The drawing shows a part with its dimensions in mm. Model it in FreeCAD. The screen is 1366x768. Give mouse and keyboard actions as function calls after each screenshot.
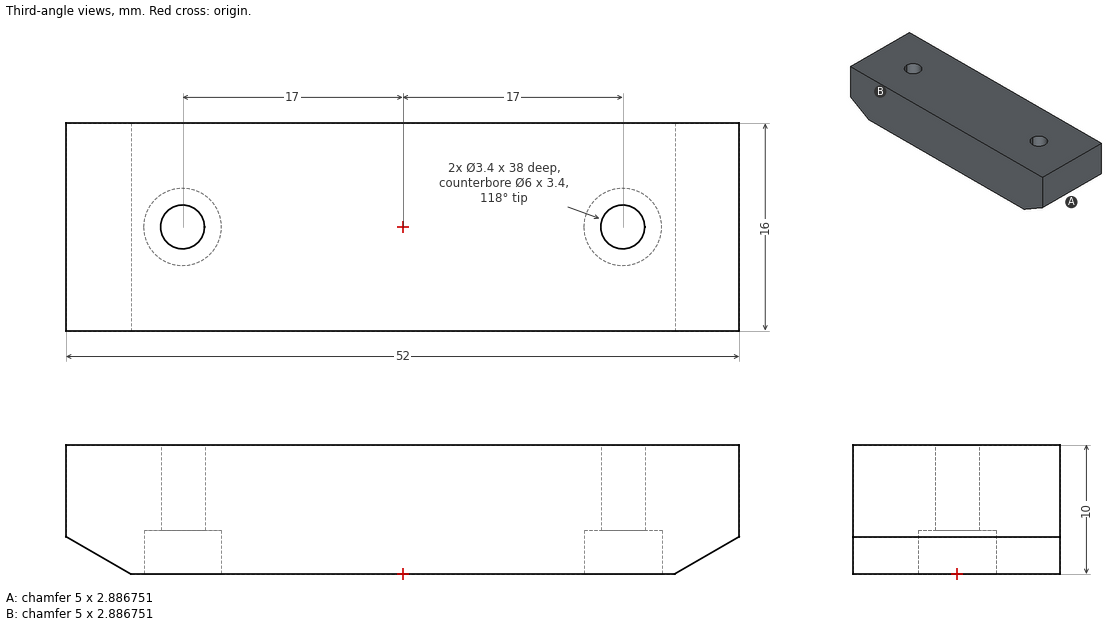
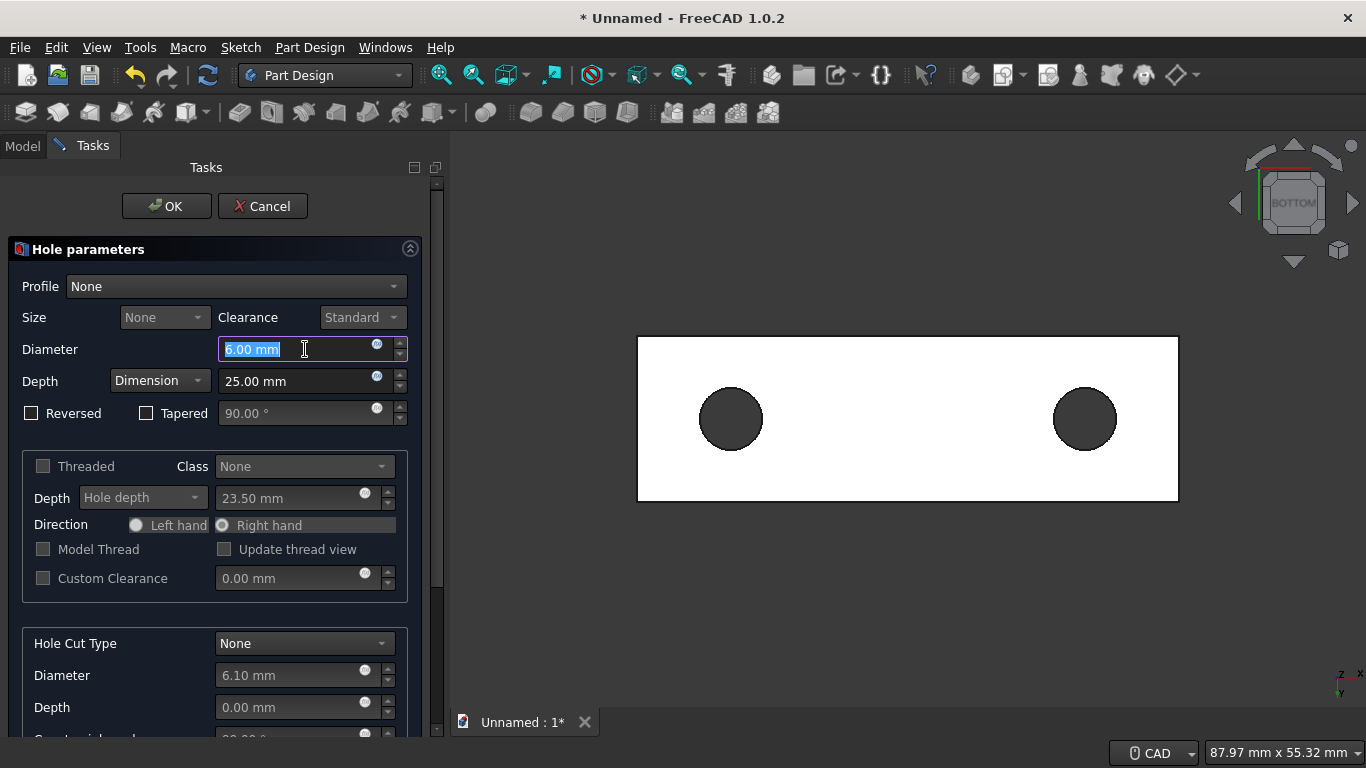
text(3.4)
key(Tab)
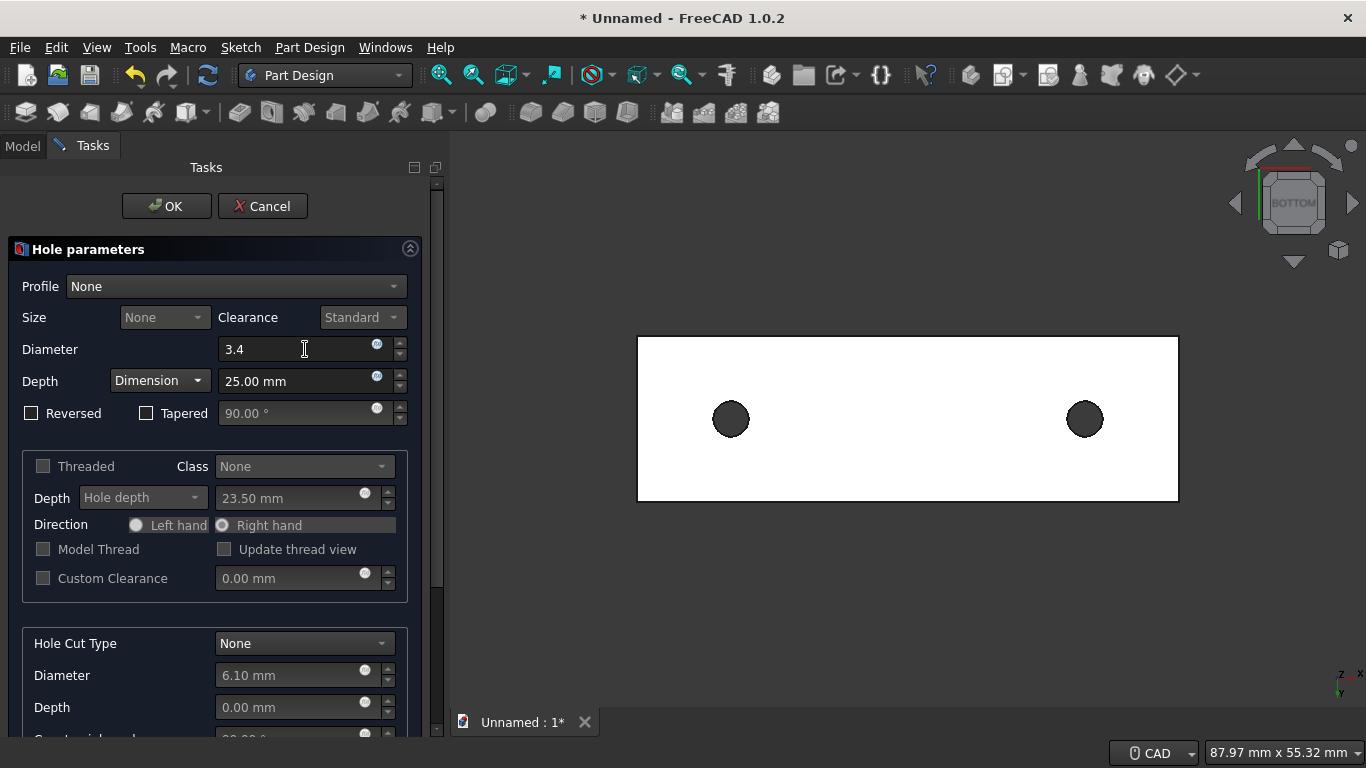
triple_click(305, 381)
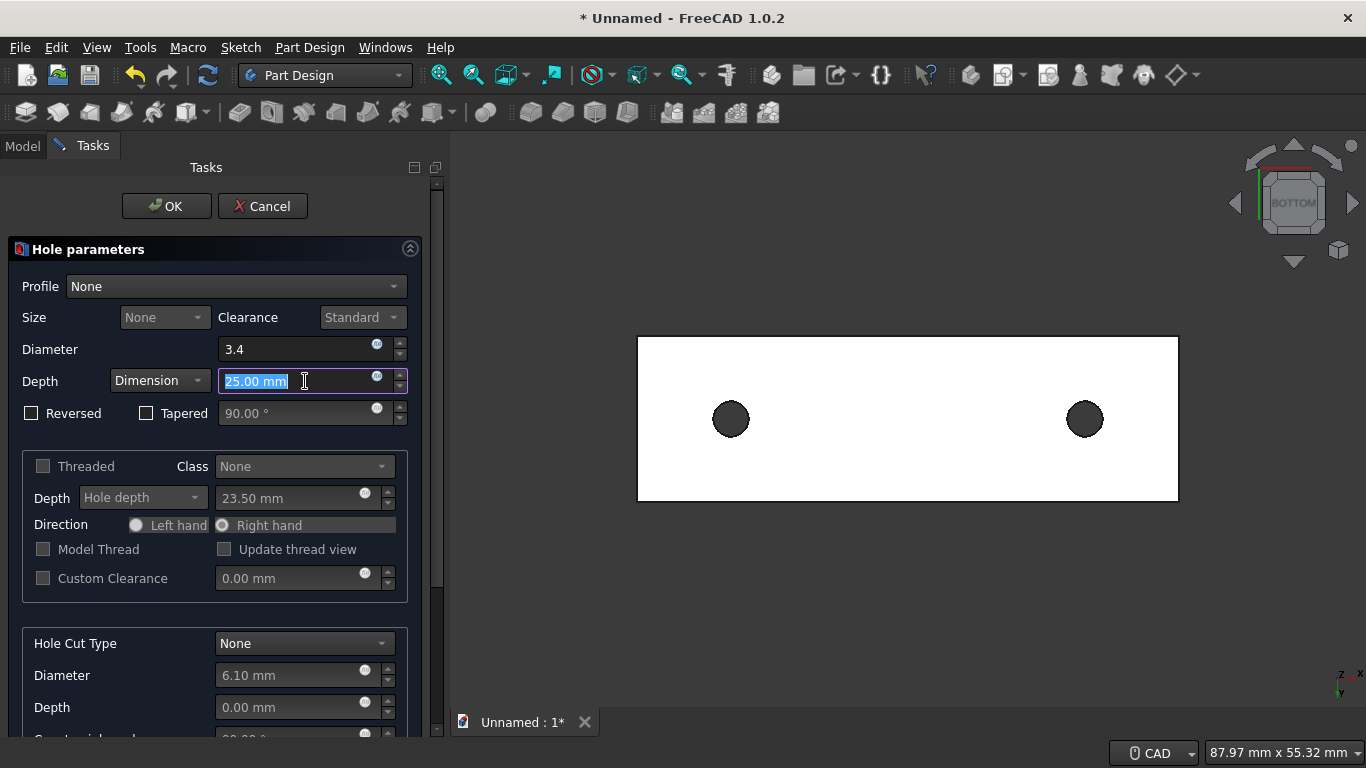
text(38)
key(Tab)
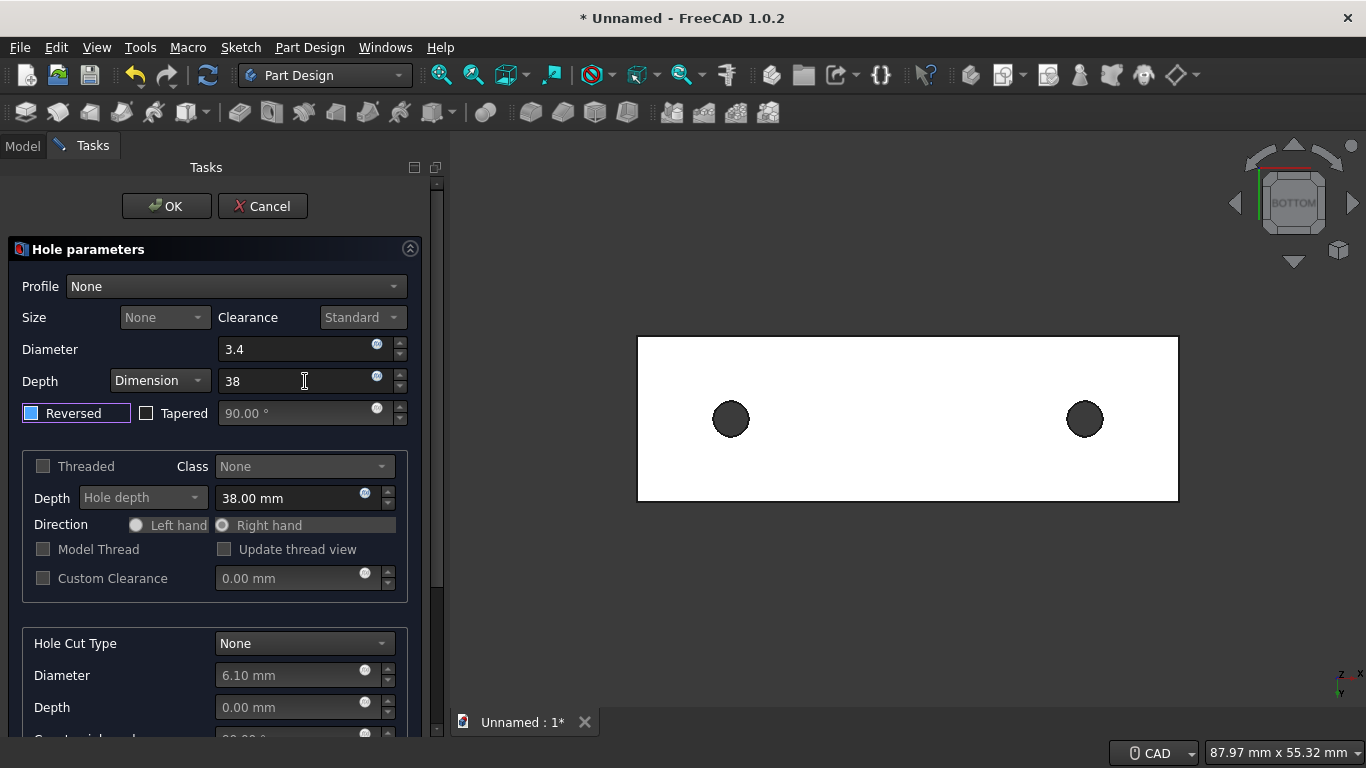
click(306, 644)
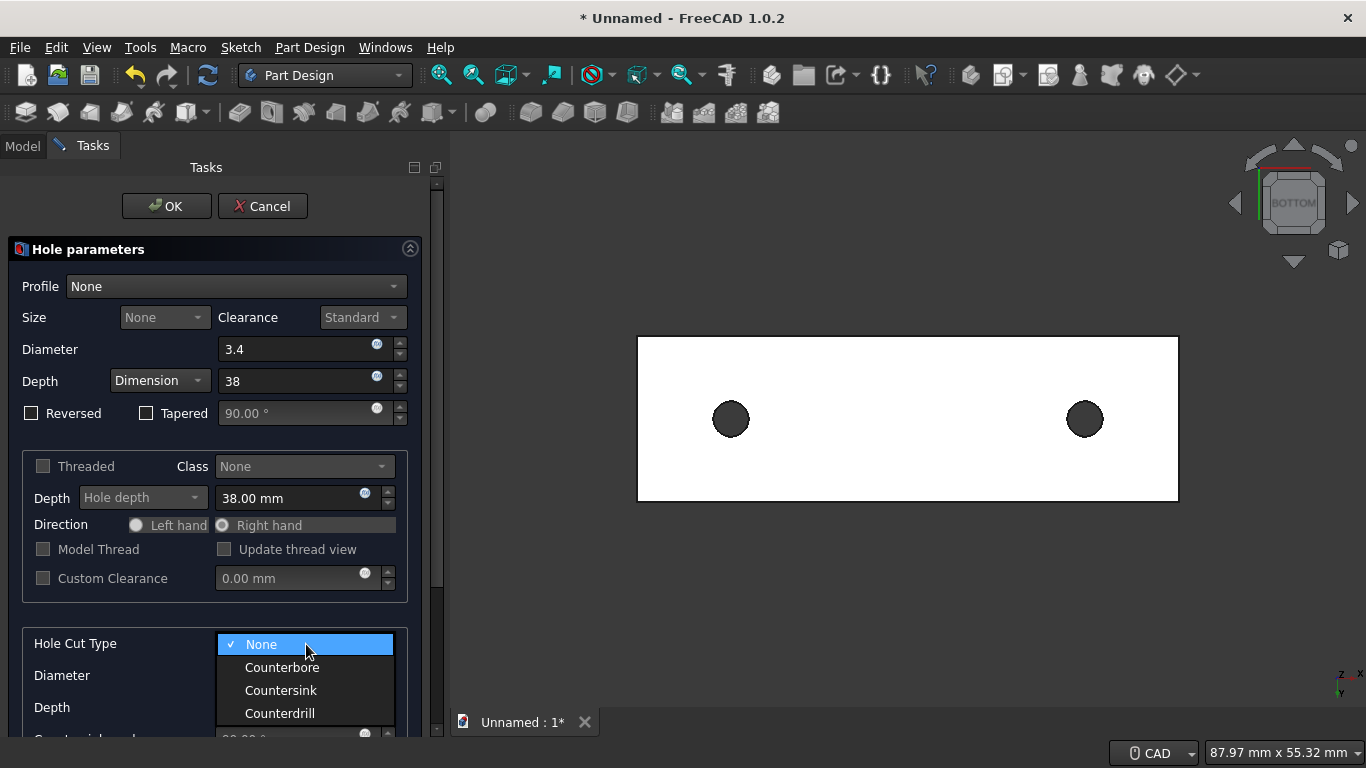
click(304, 668)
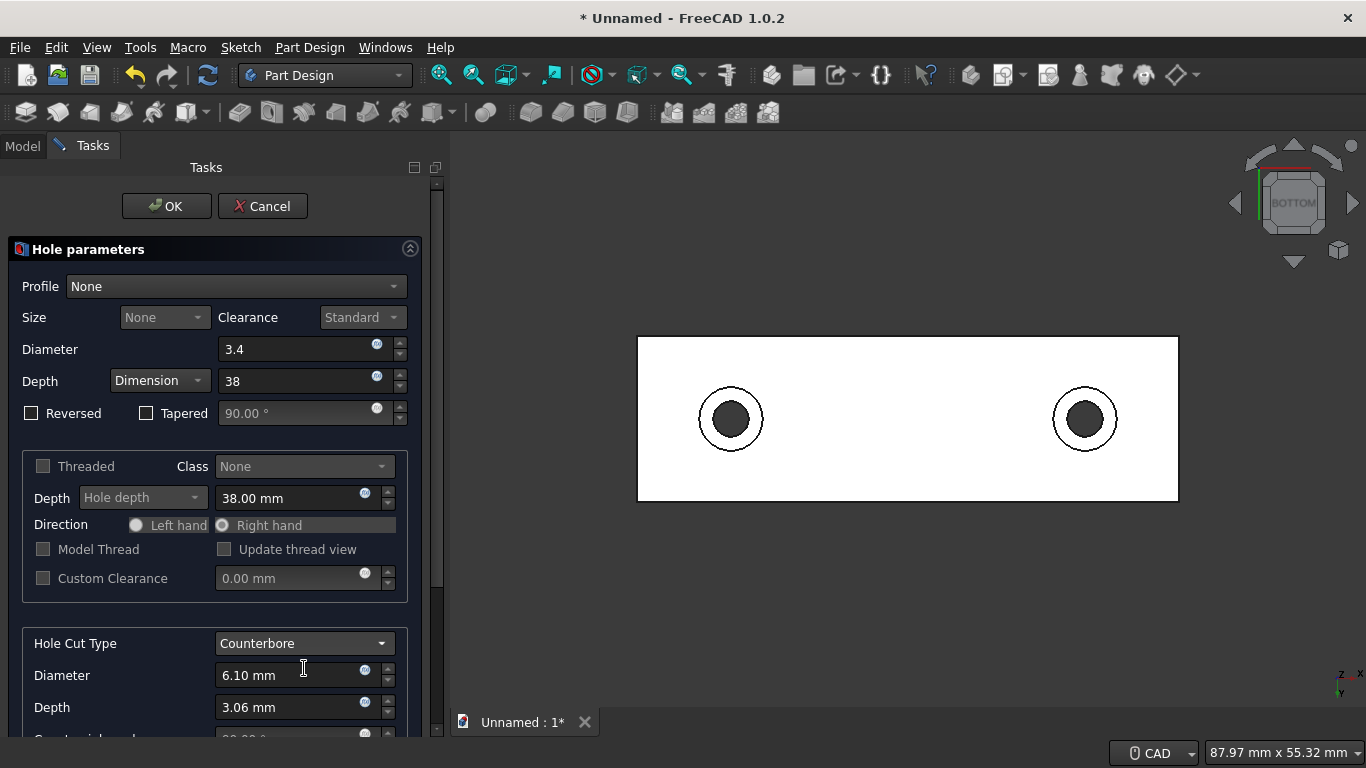
triple_click(298, 675)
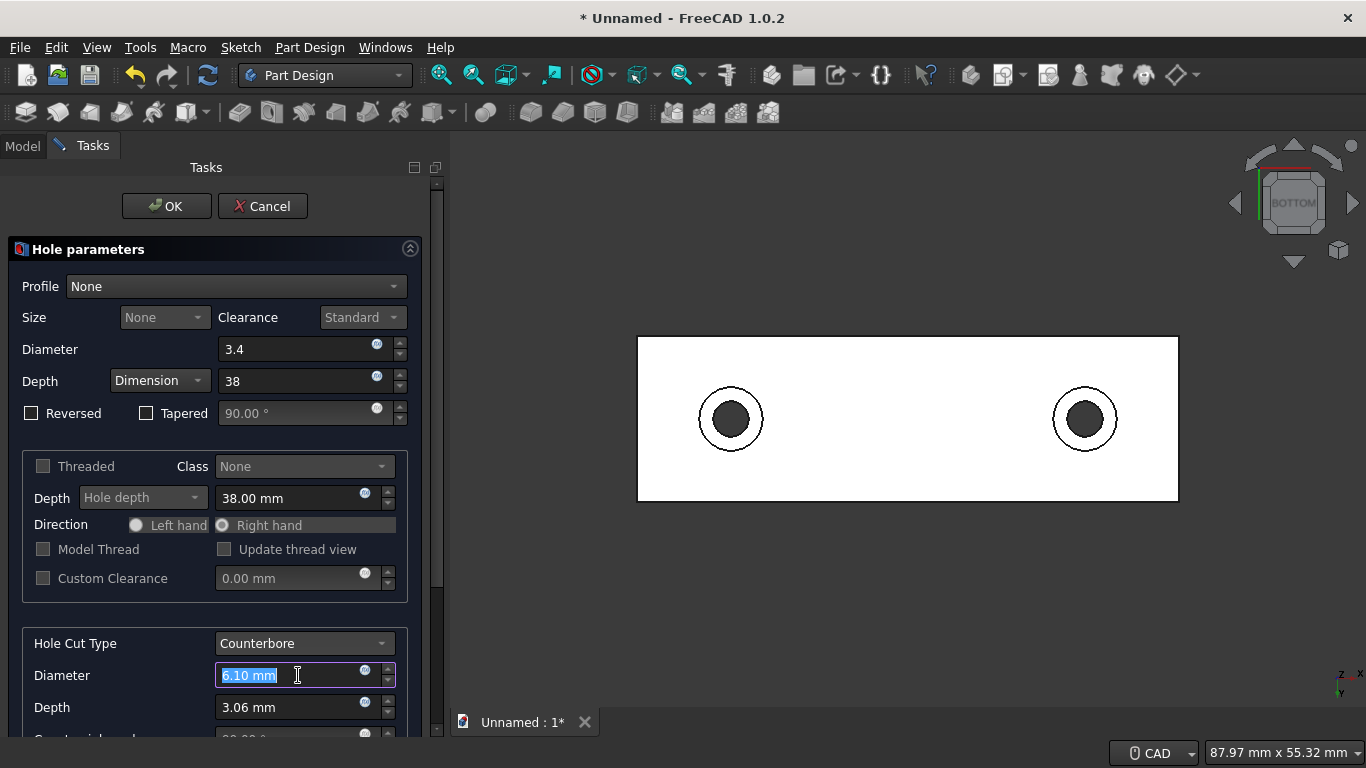
text(6)
key(Tab)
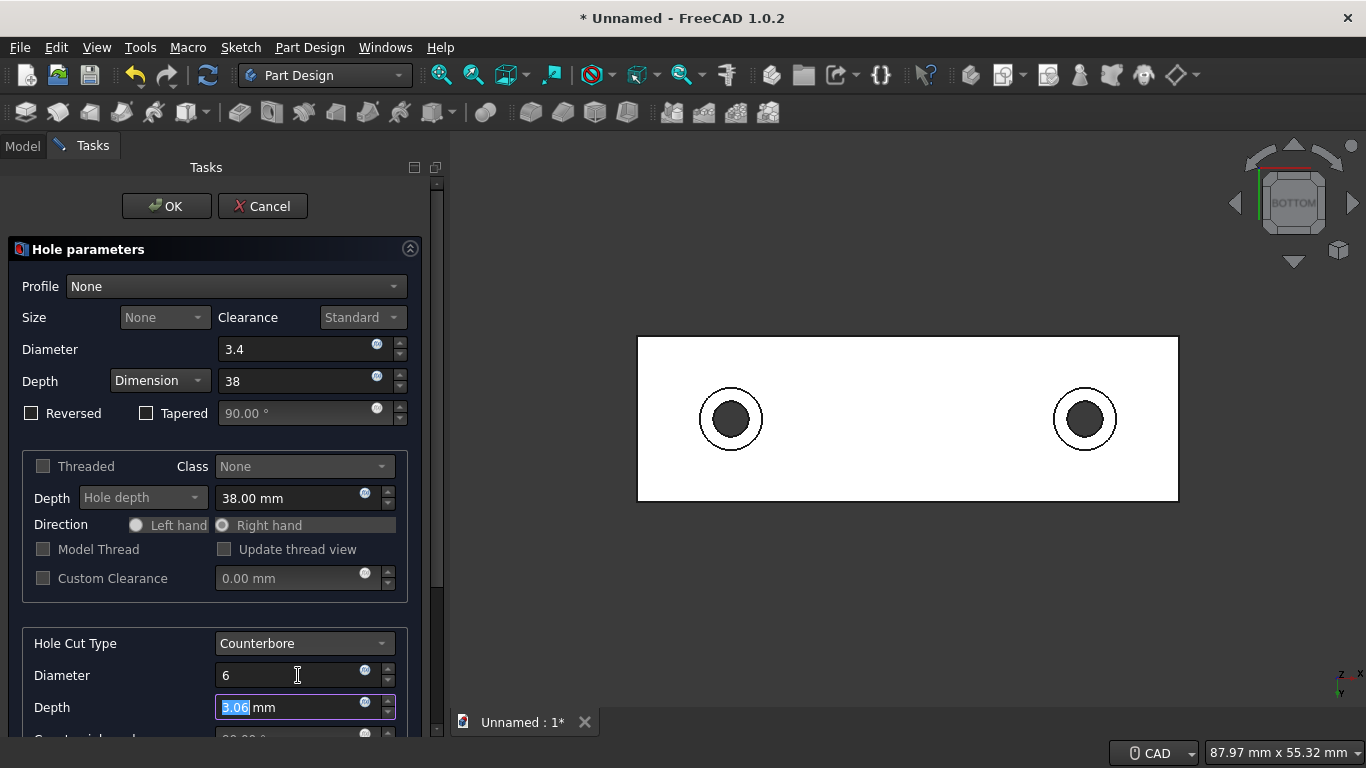
text(3.4)
key(Tab)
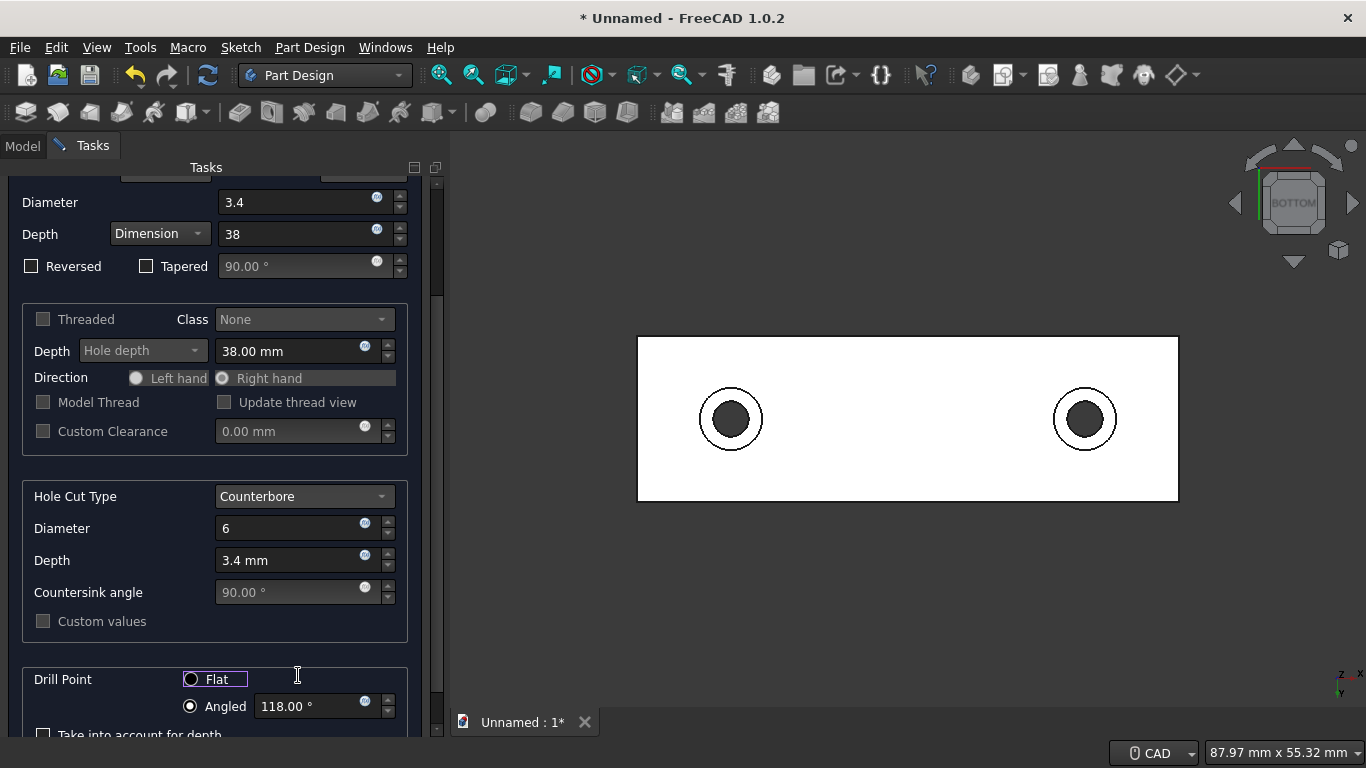
scroll(437, 456, up, 4)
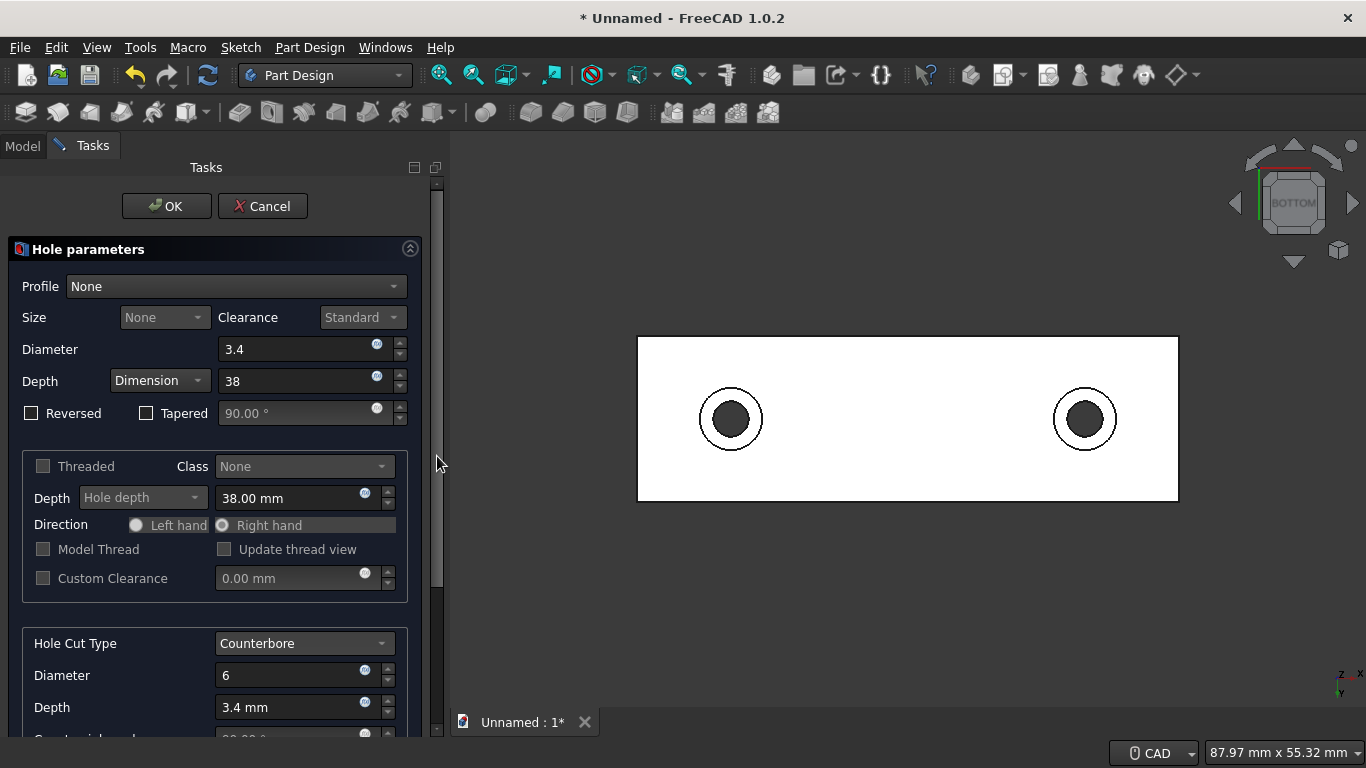
click(167, 206)